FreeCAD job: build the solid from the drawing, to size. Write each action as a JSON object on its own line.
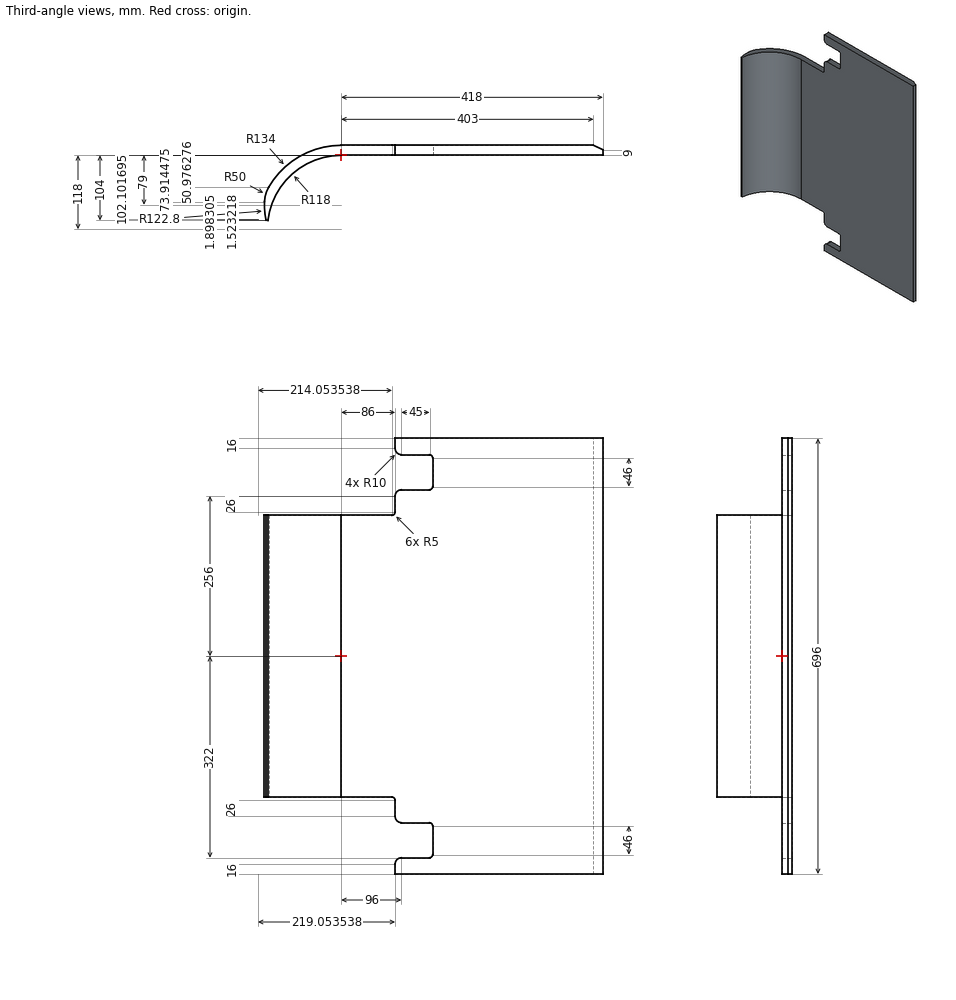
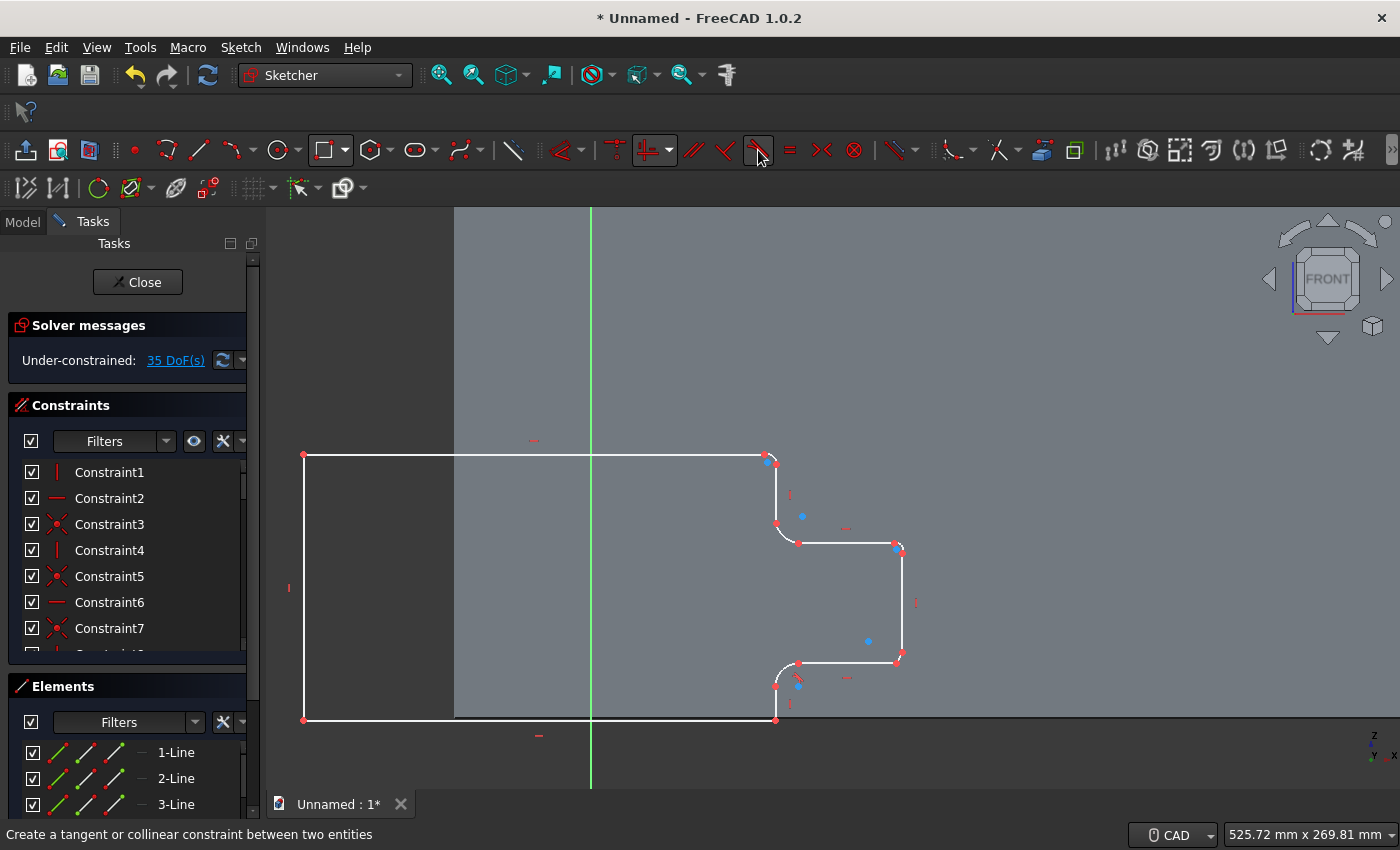
{"action": "left_click", "coordinate": [867, 663]}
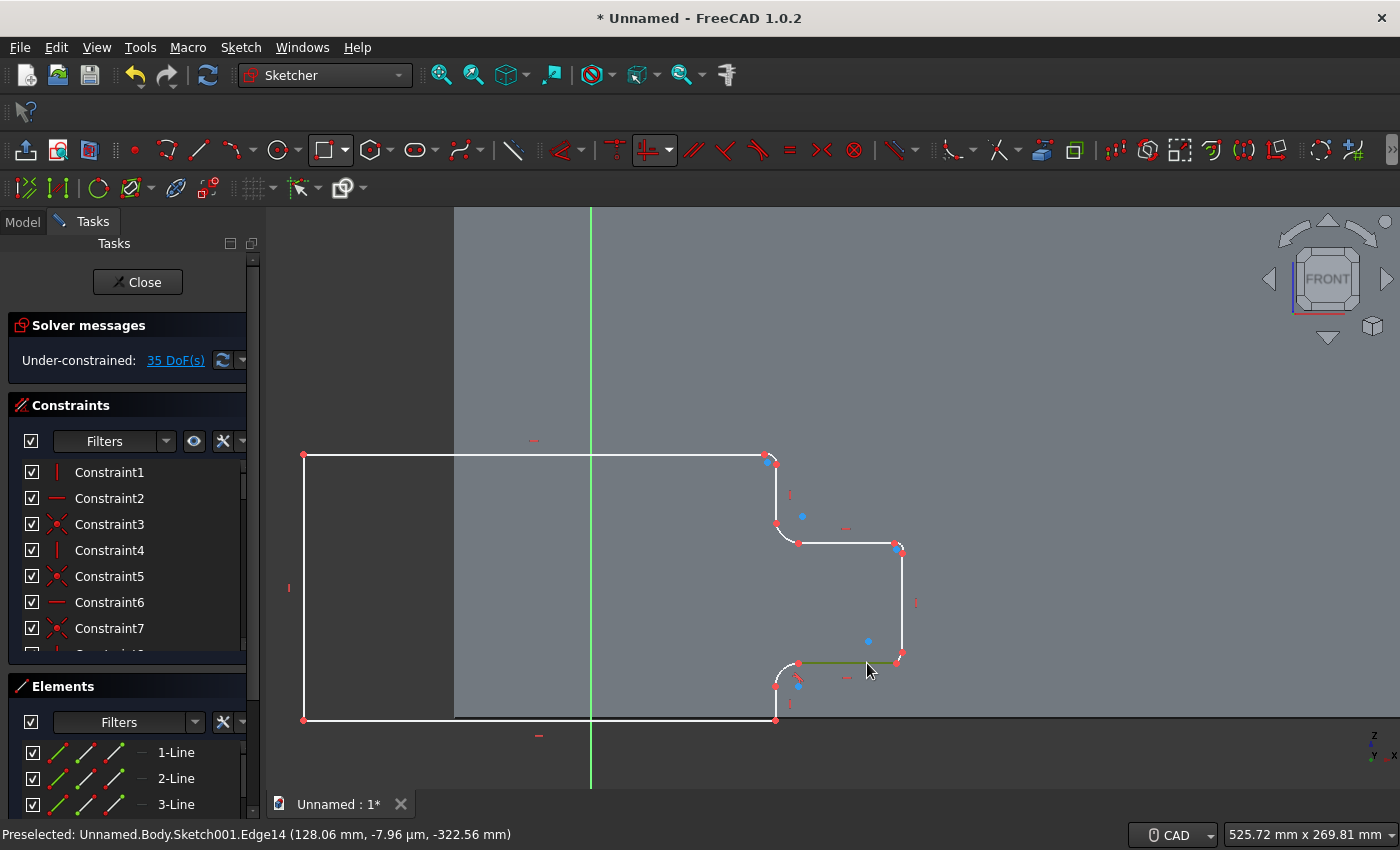
{"action": "scroll", "coordinate": [900, 658], "scroll_direction": "up", "scroll_amount": 4}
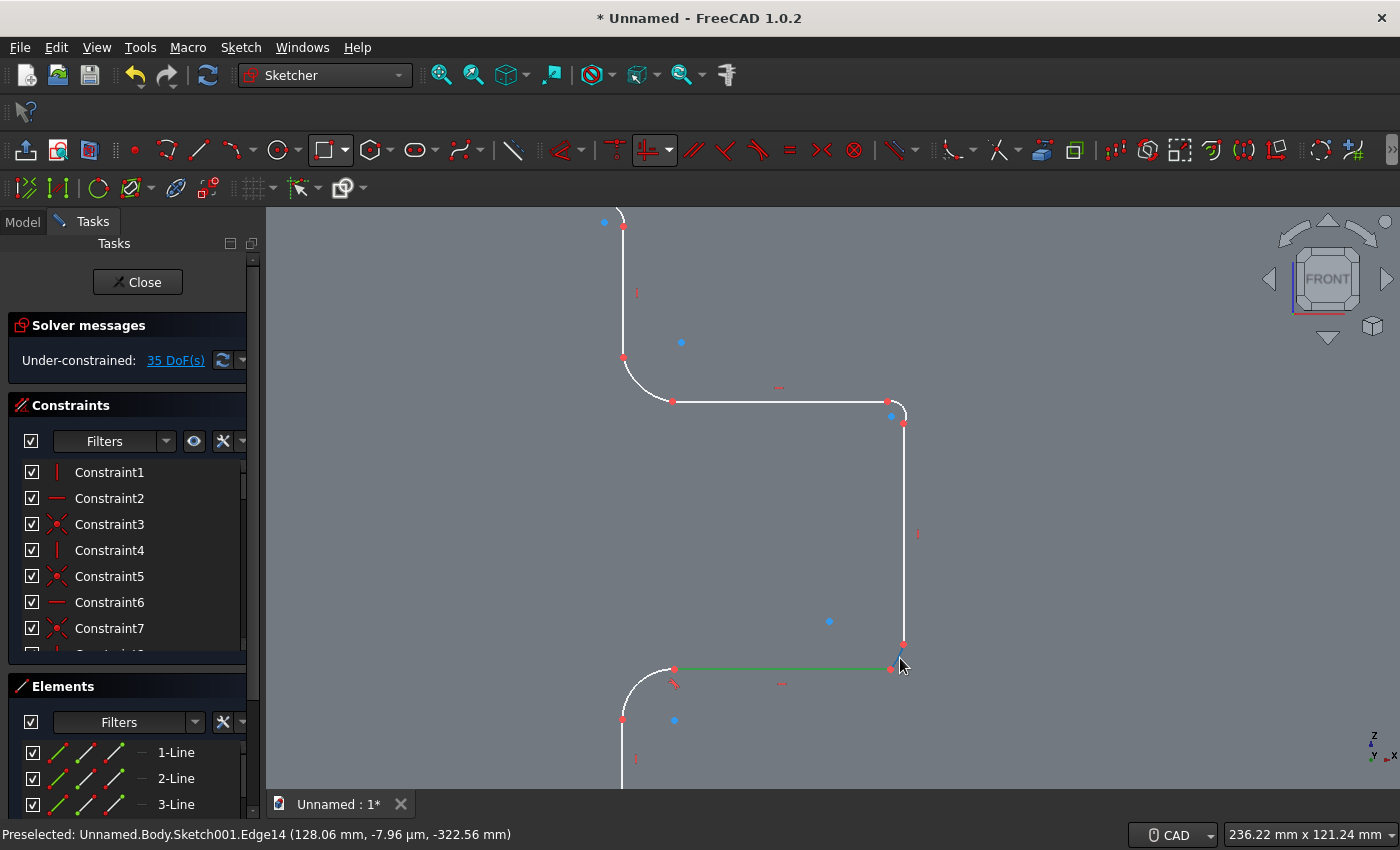
{"action": "left_click", "coordinate": [898, 657]}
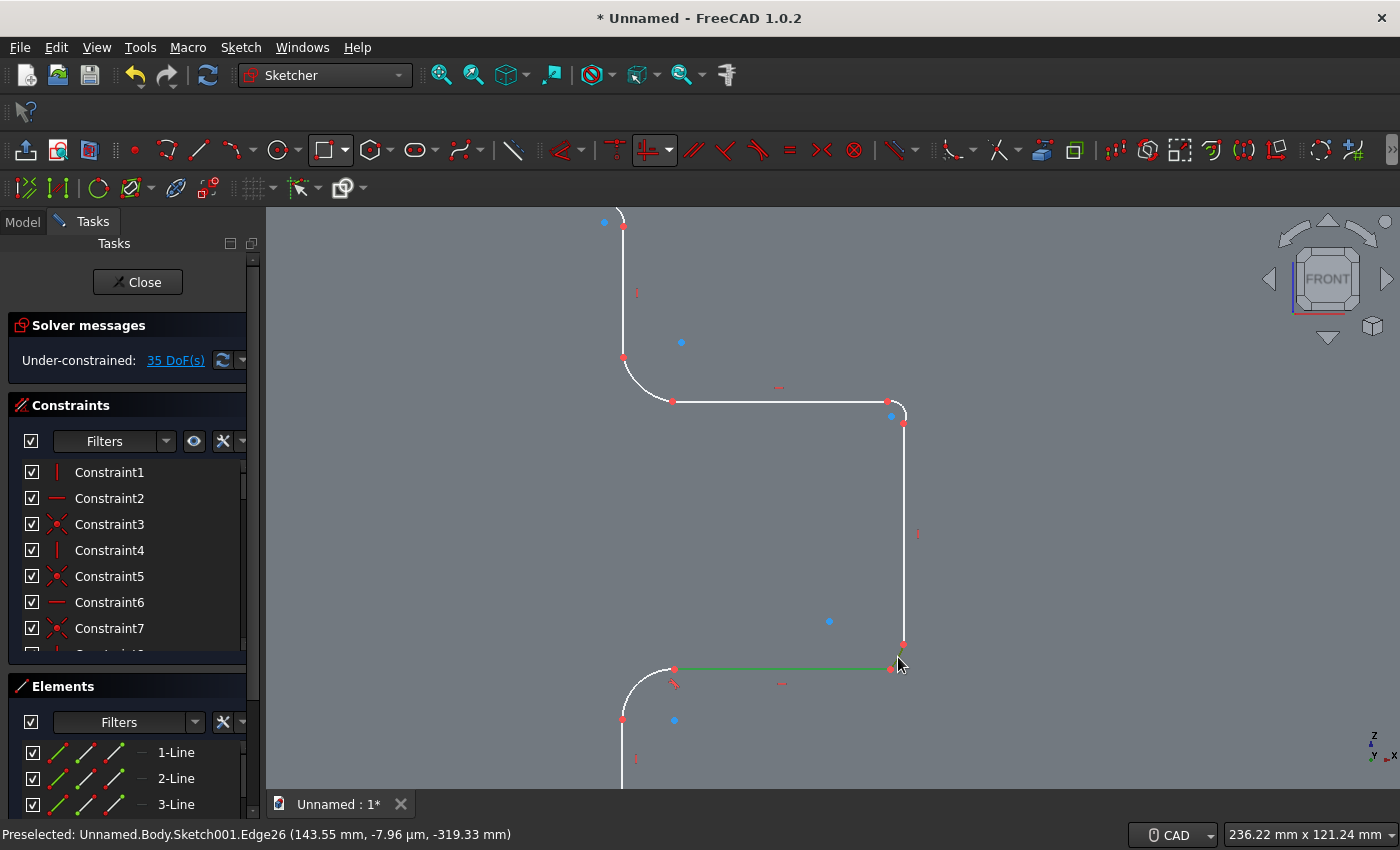
{"action": "left_click", "coordinate": [758, 150]}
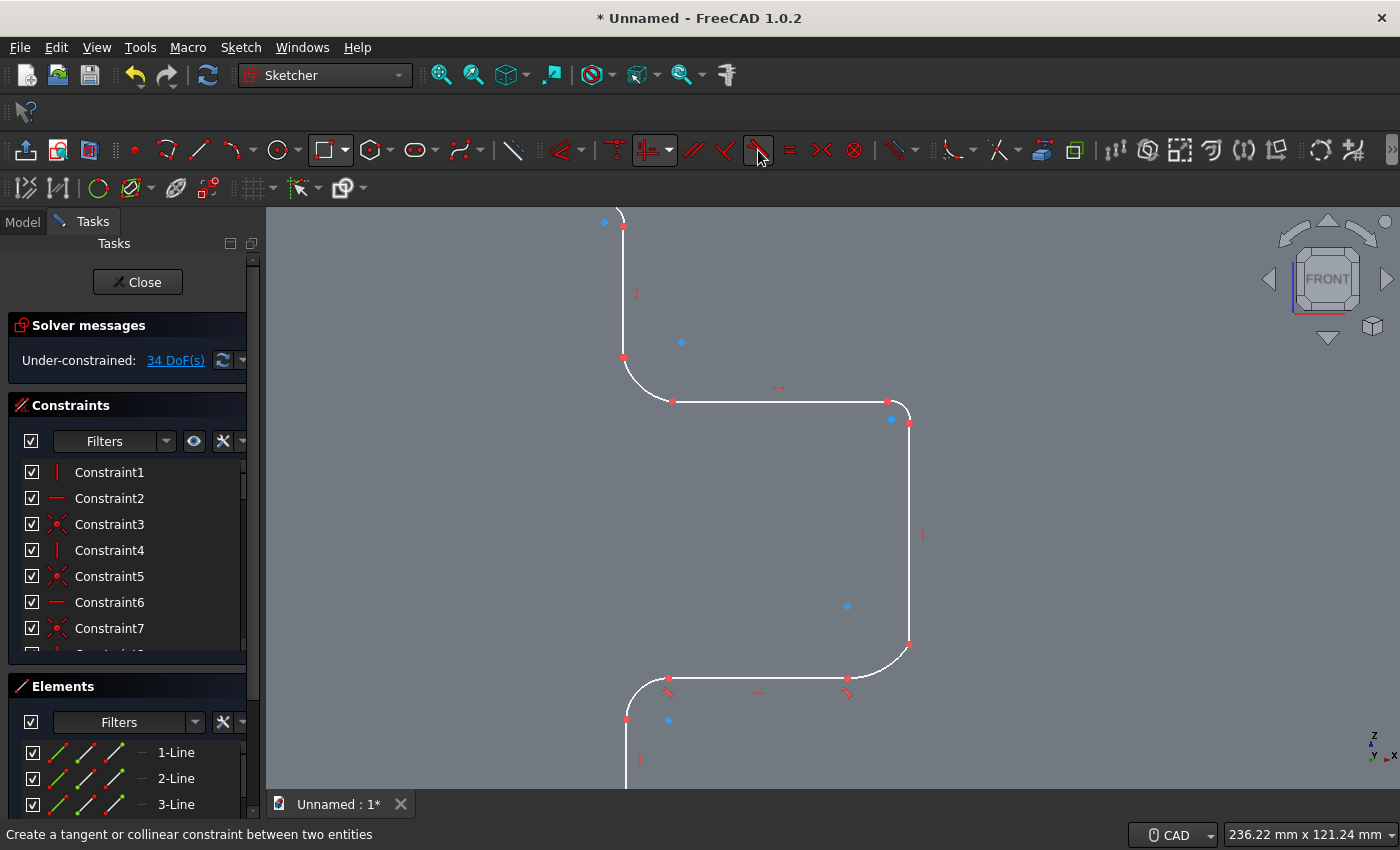
{"action": "left_click", "coordinate": [626, 743]}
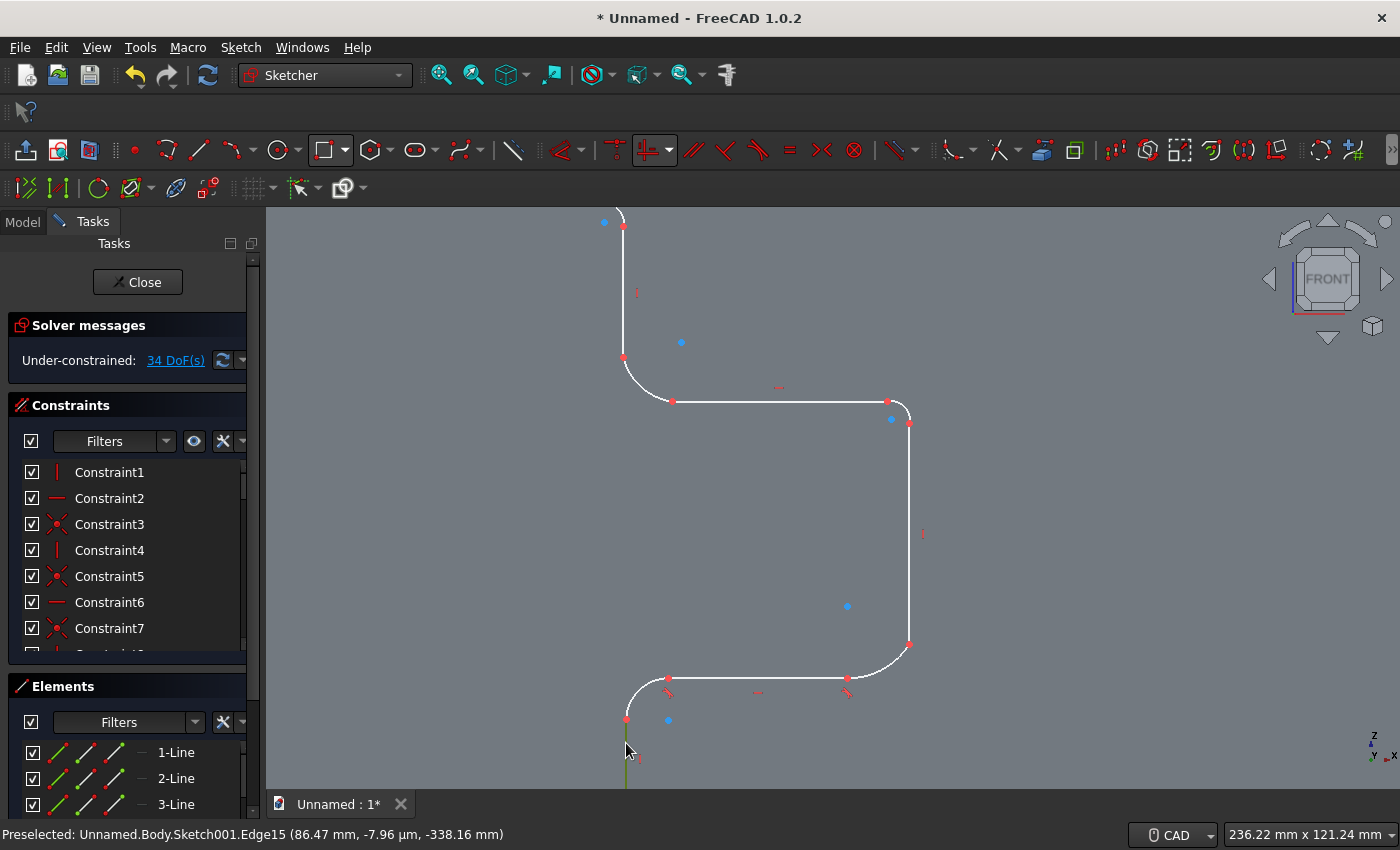
{"action": "left_click", "coordinate": [650, 683]}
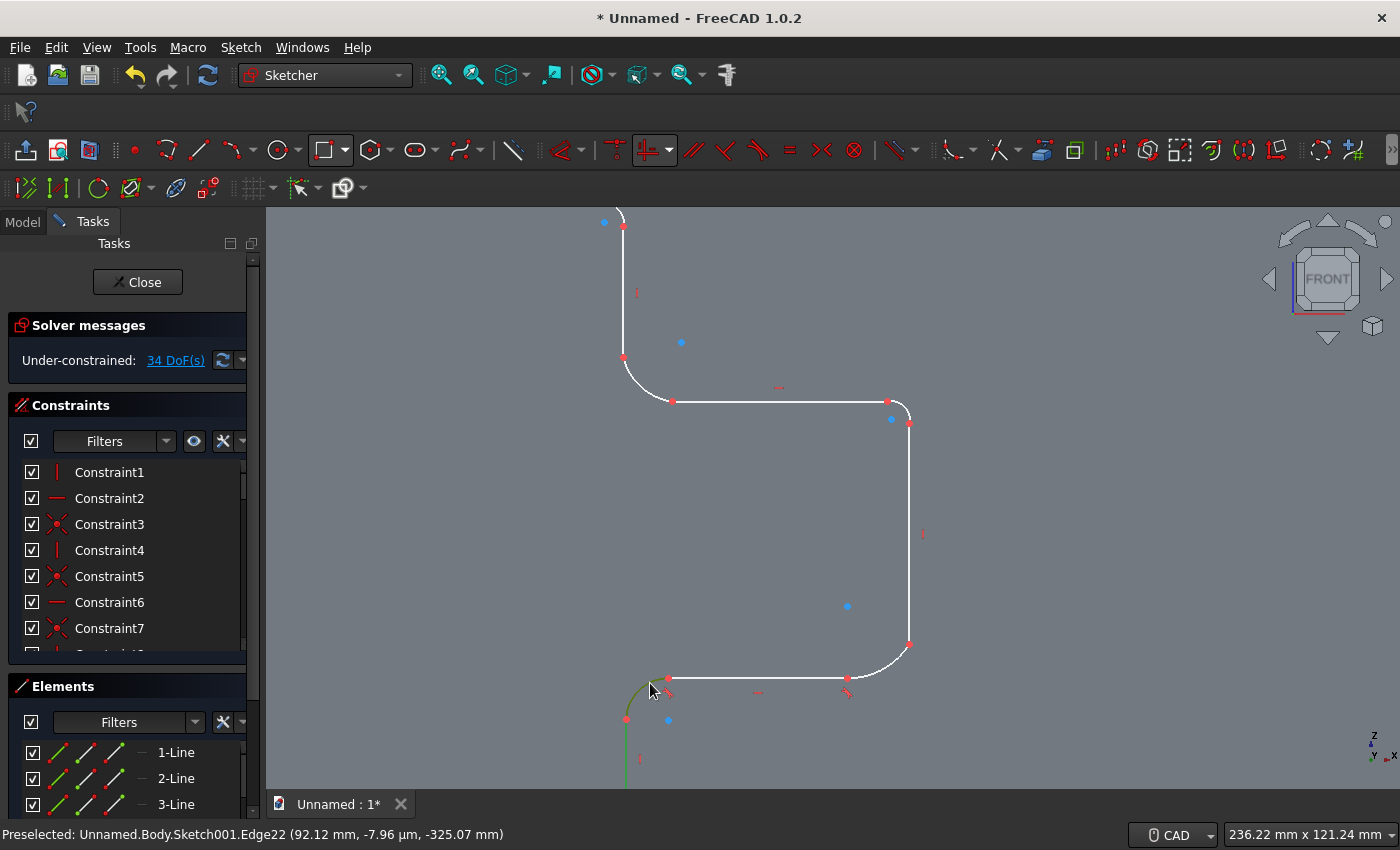
{"action": "left_click", "coordinate": [758, 150]}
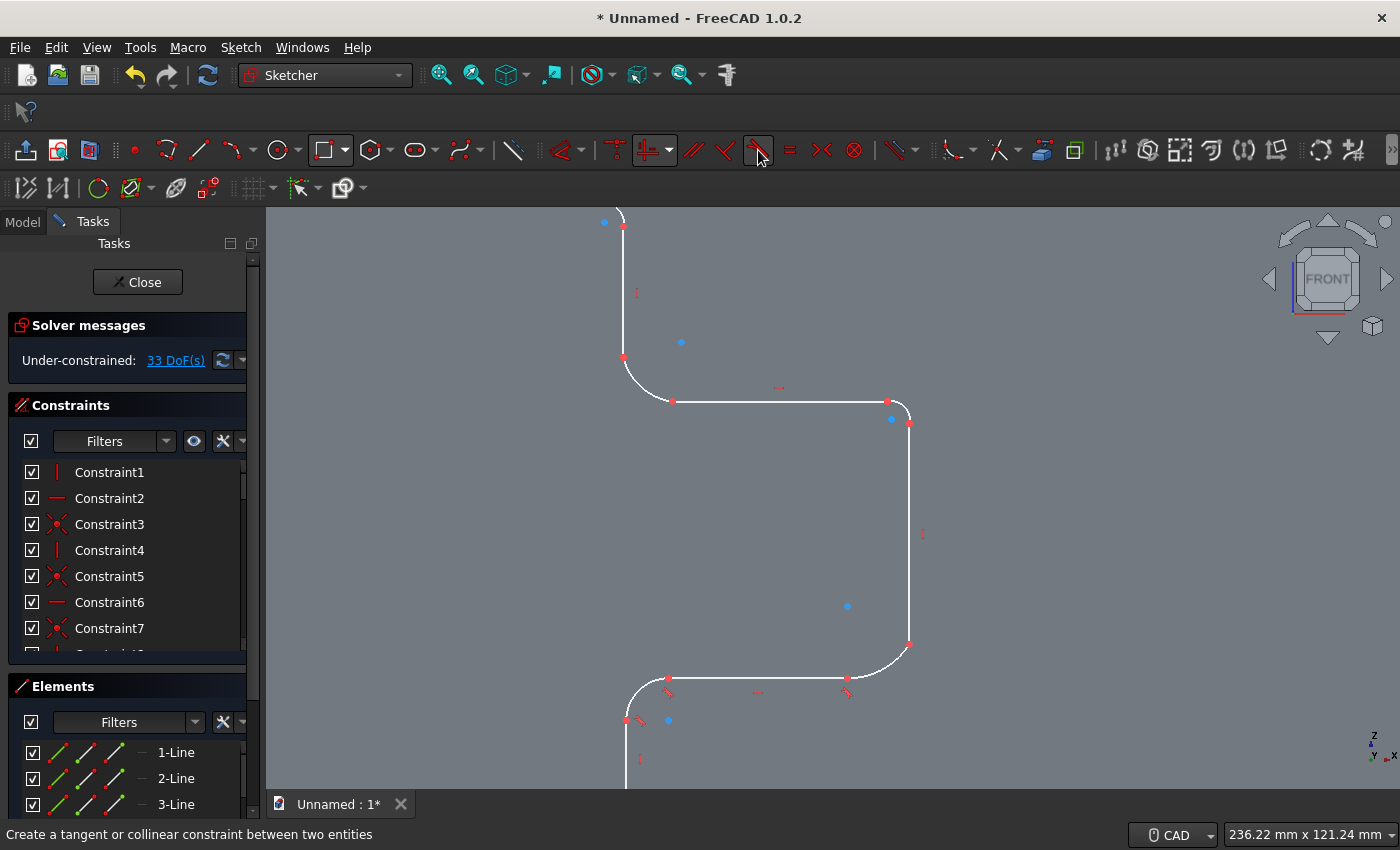
{"action": "scroll", "coordinate": [830, 670], "scroll_direction": "down", "scroll_amount": 11}